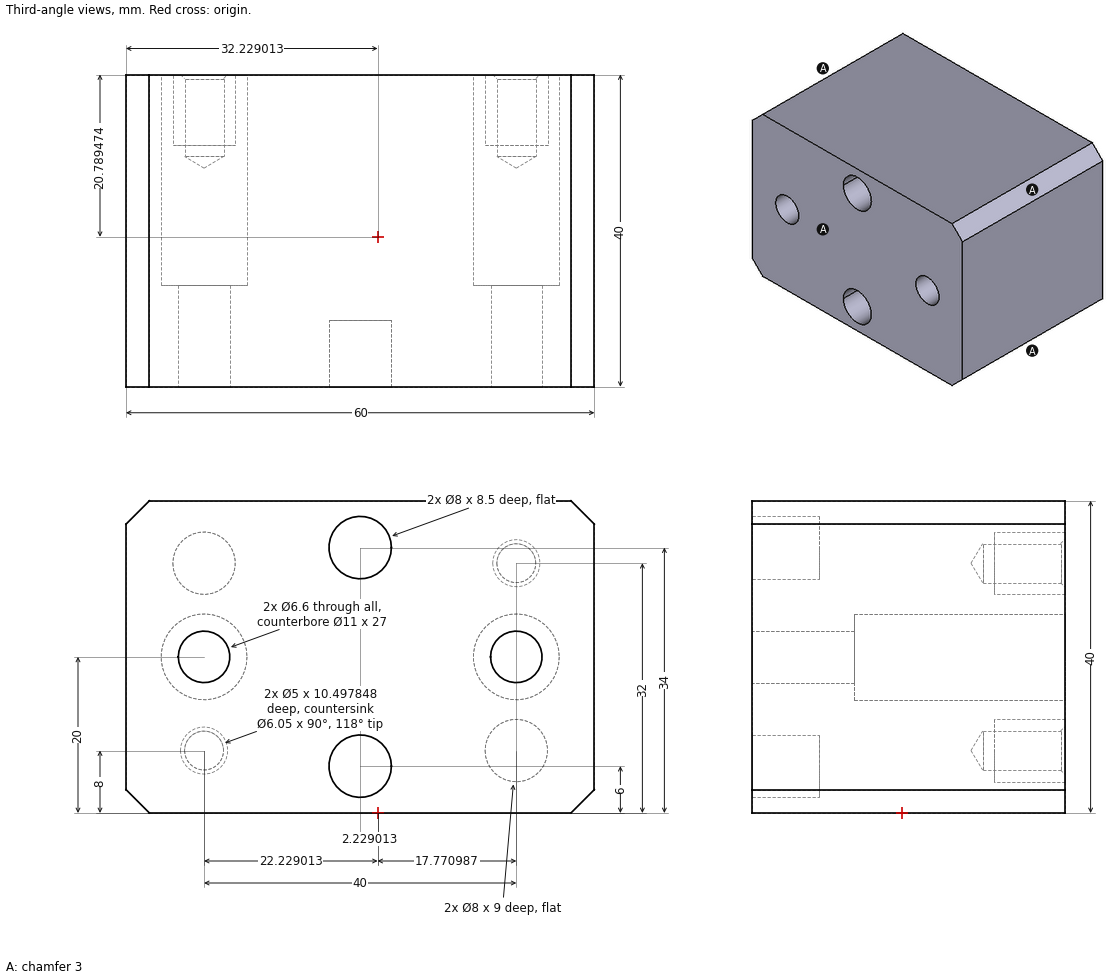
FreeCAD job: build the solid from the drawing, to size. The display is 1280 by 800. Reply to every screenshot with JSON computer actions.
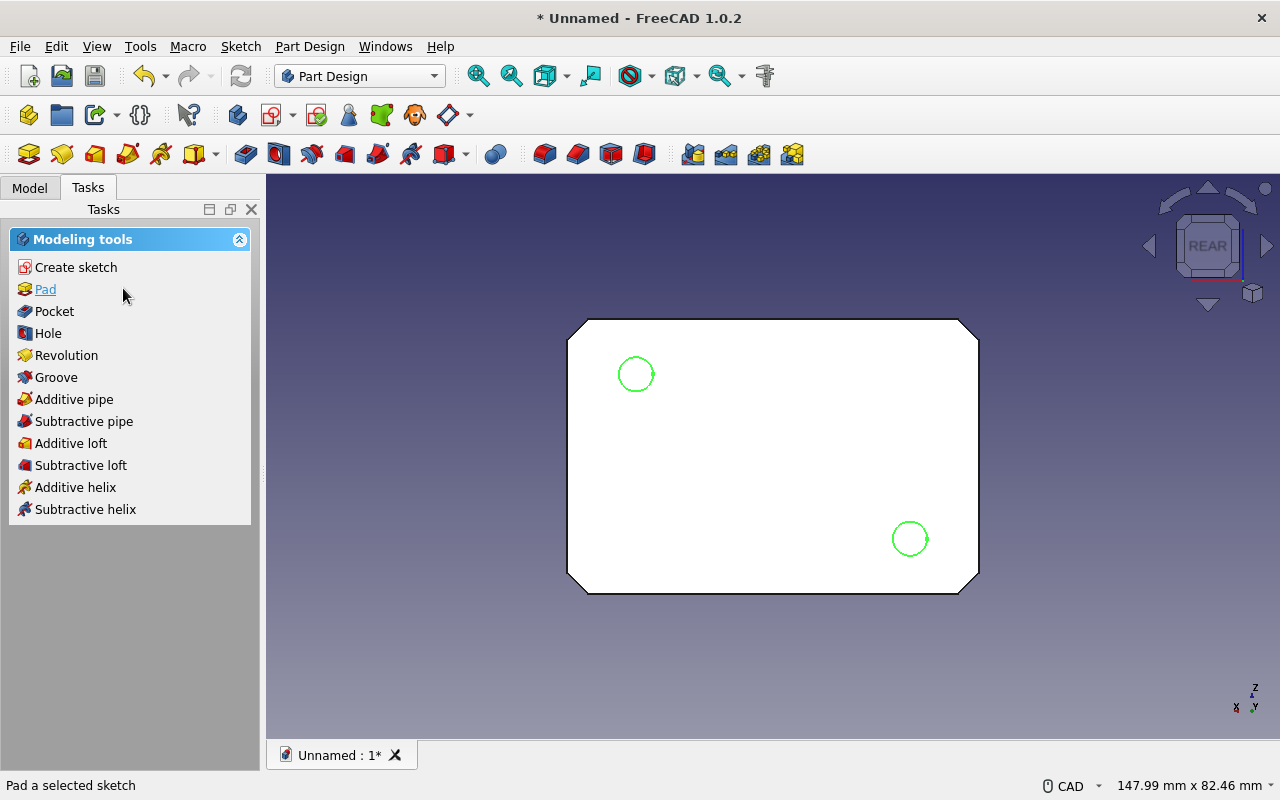
{"action": "left_click", "coordinate": [279, 154]}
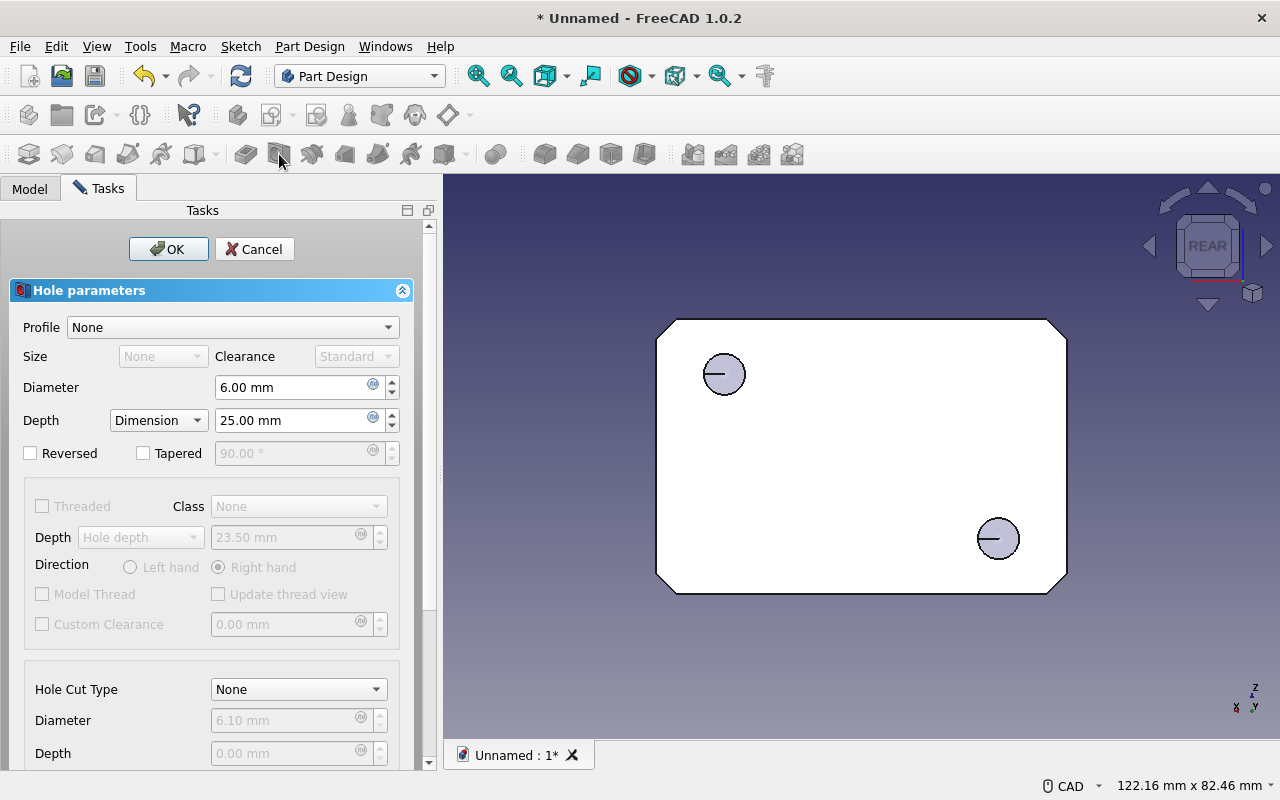
{"action": "triple_click", "coordinate": [300, 388]}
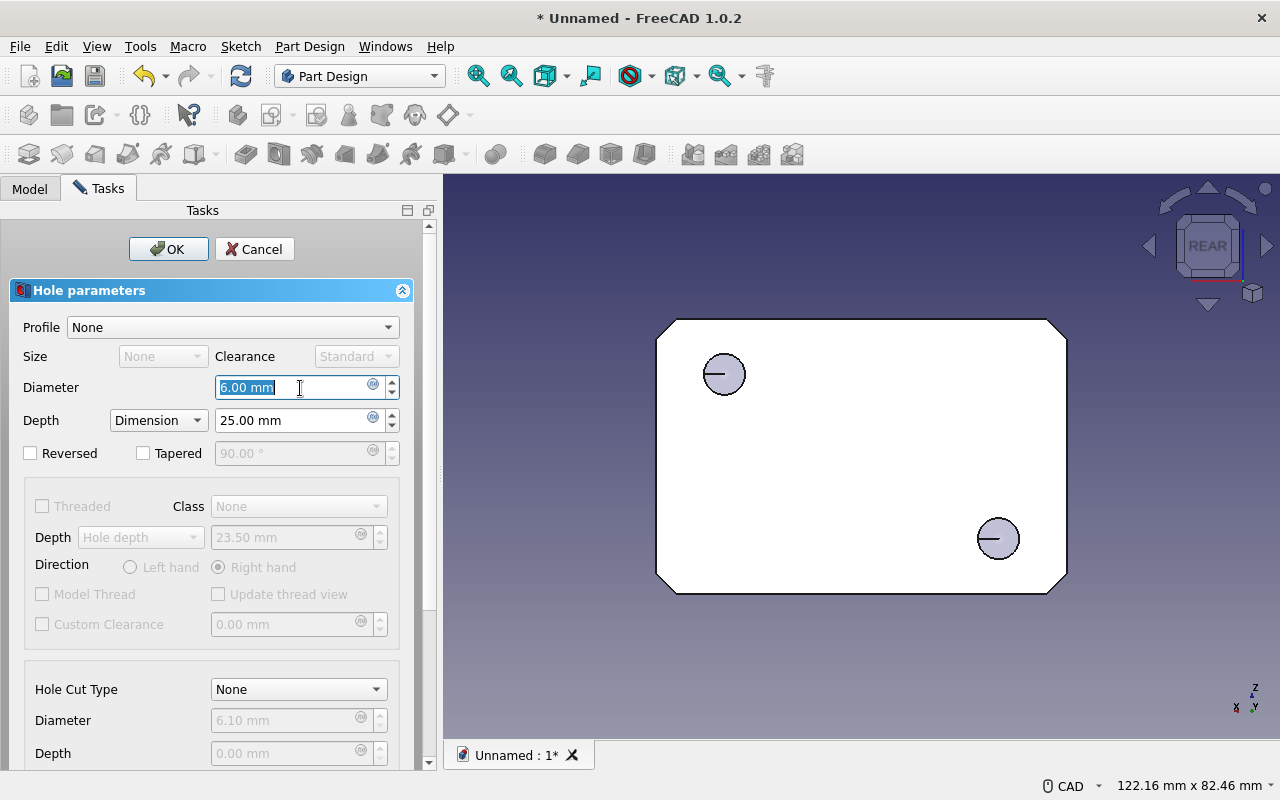
{"action": "type", "text": "5"}
{"action": "key", "text": "Tab"}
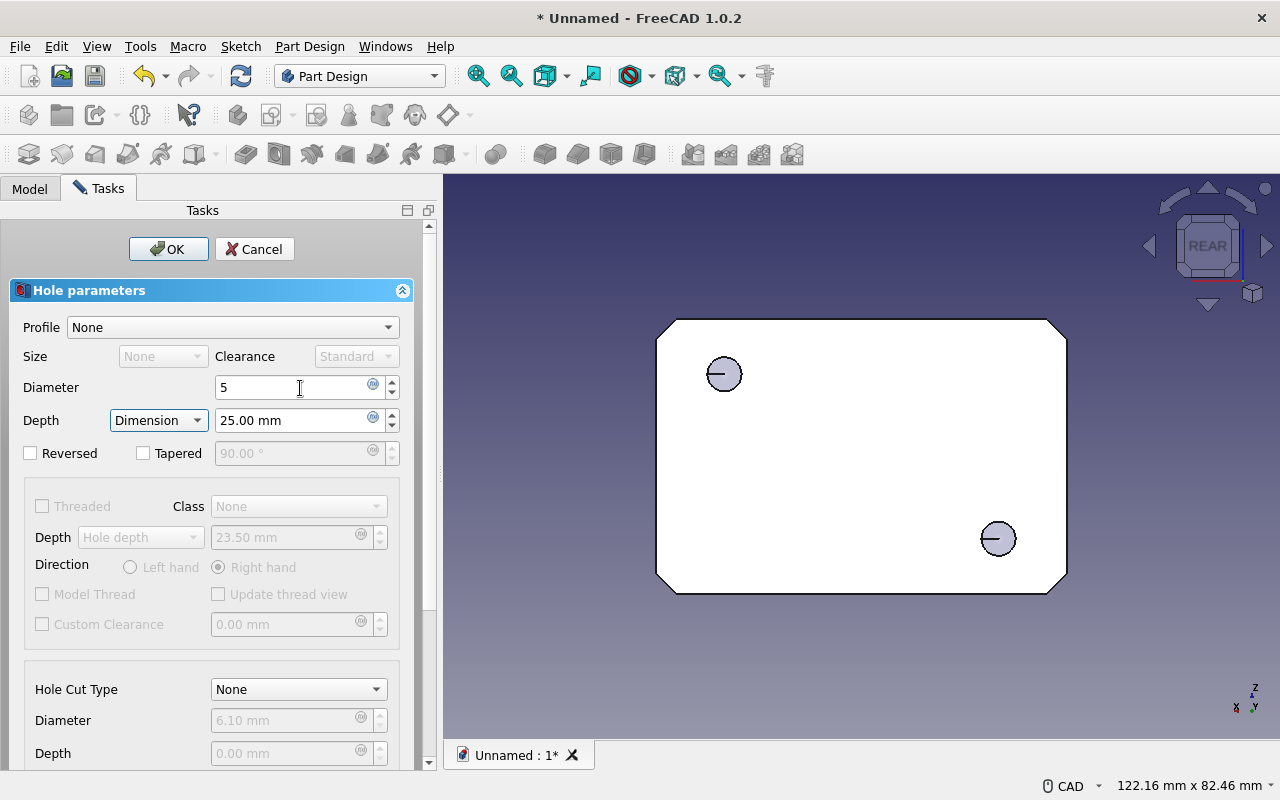
{"action": "triple_click", "coordinate": [300, 420]}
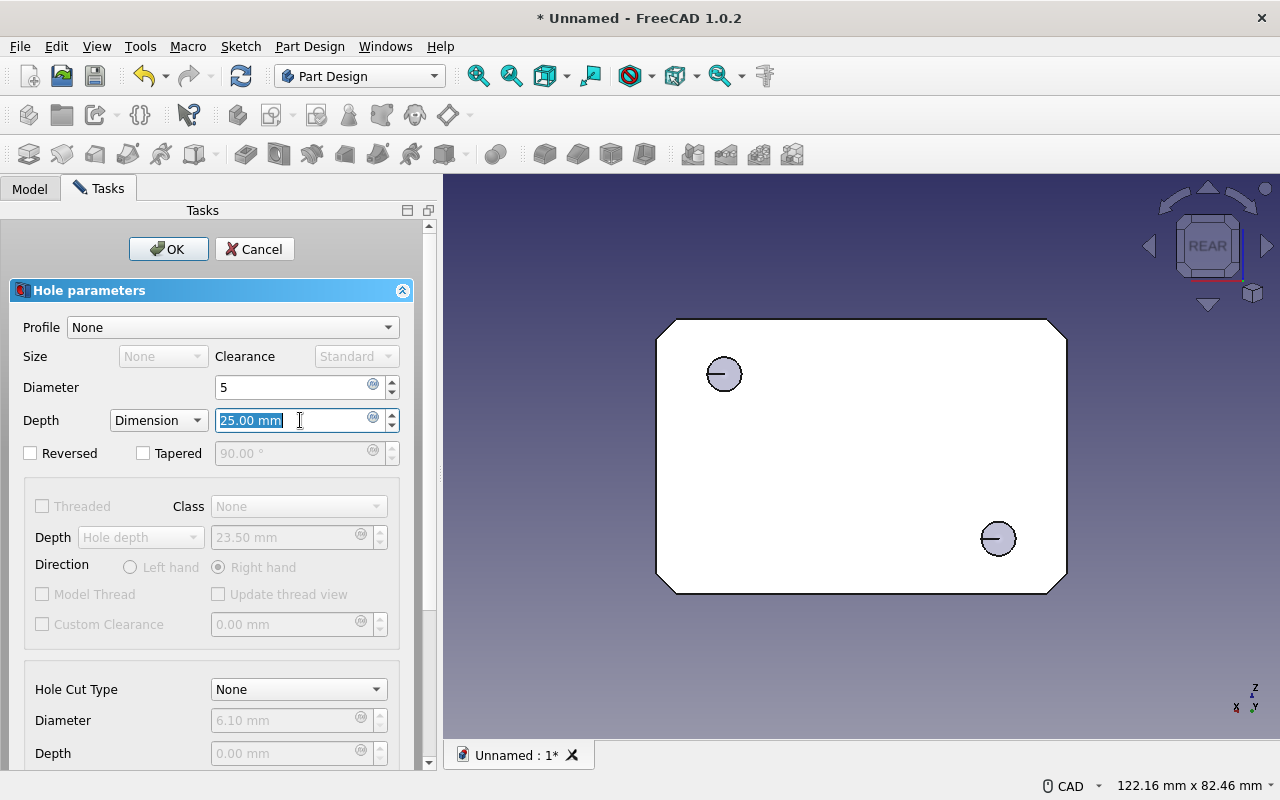
{"action": "type", "text": "10.497848"}
{"action": "key", "text": "Tab"}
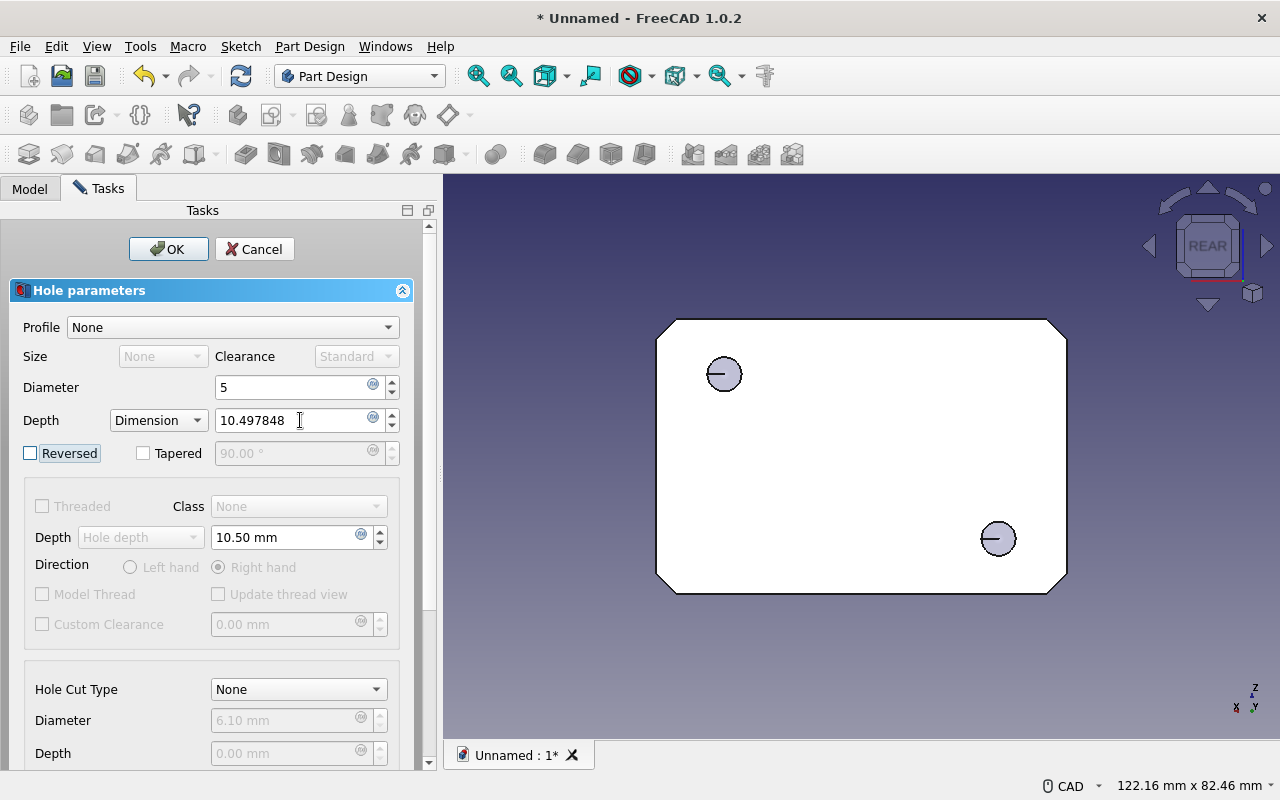
{"action": "left_click", "coordinate": [300, 690]}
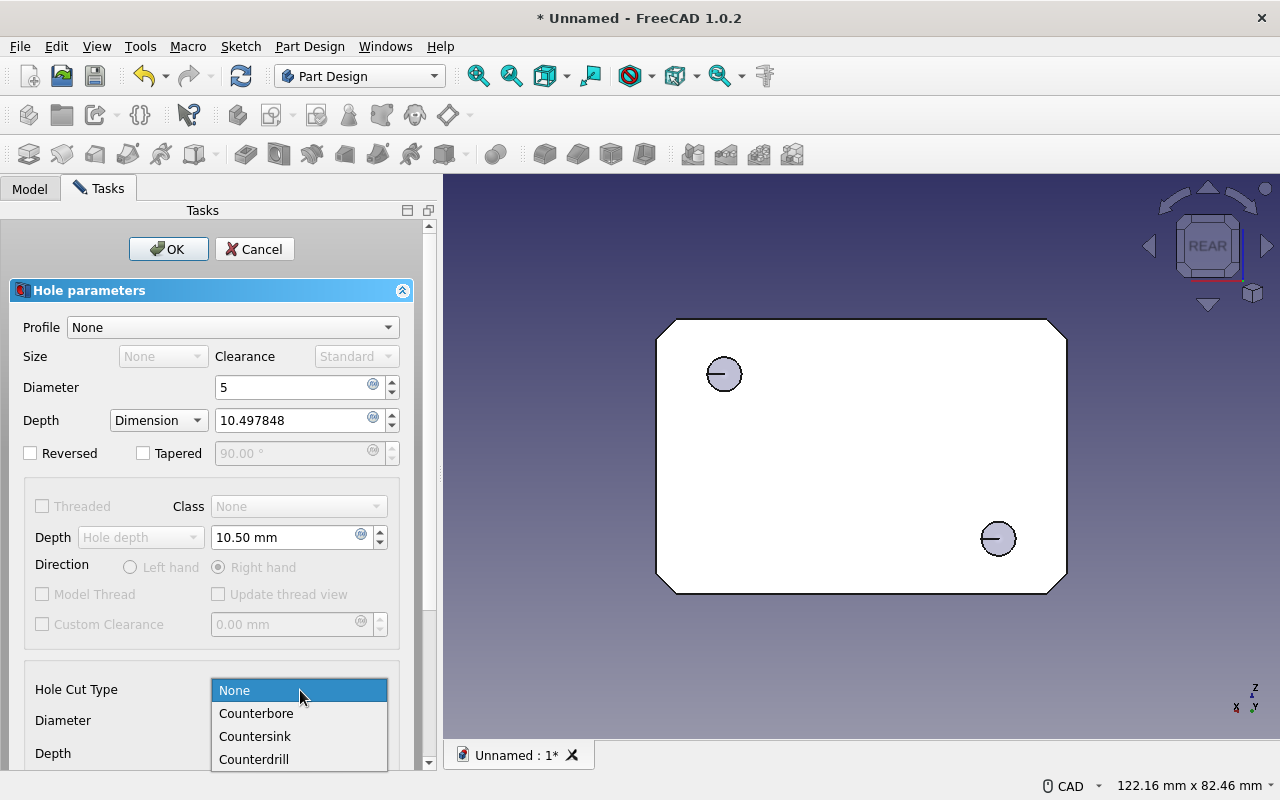
{"action": "left_click", "coordinate": [298, 736]}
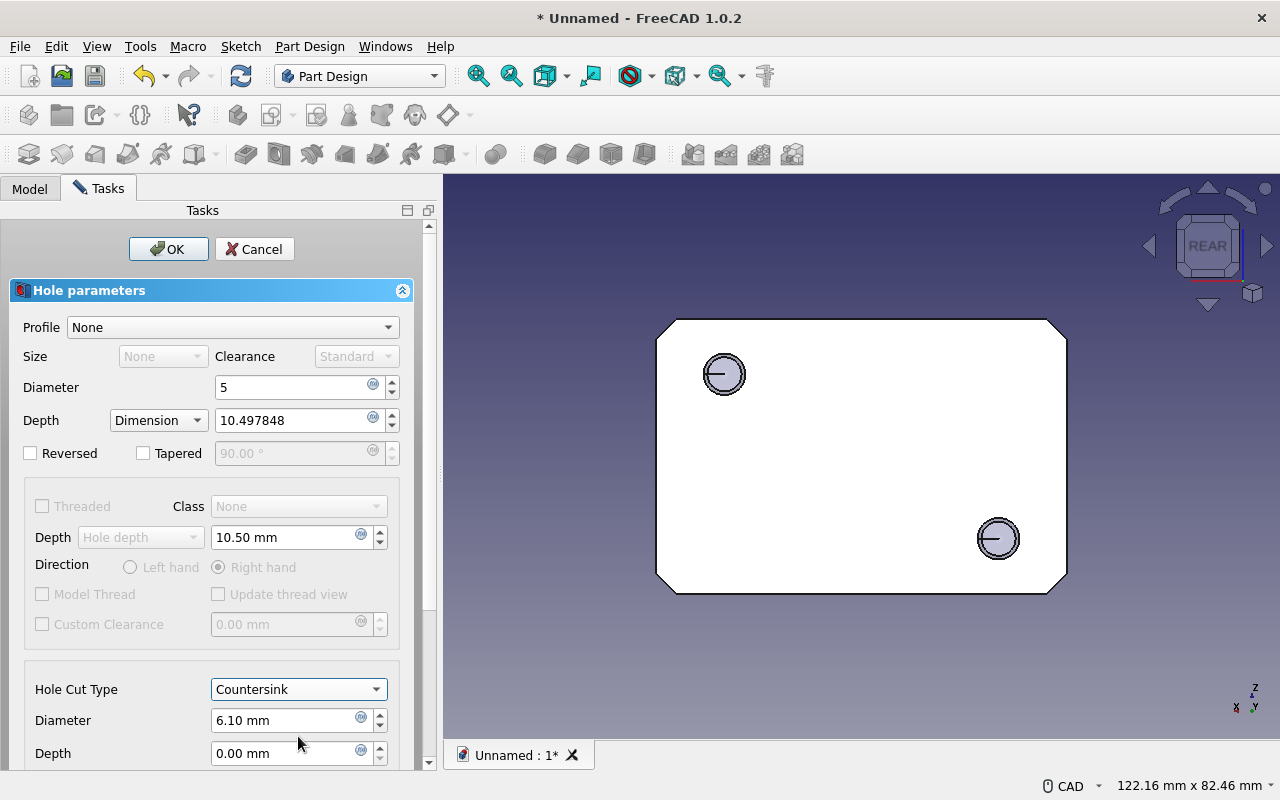
{"action": "triple_click", "coordinate": [292, 720]}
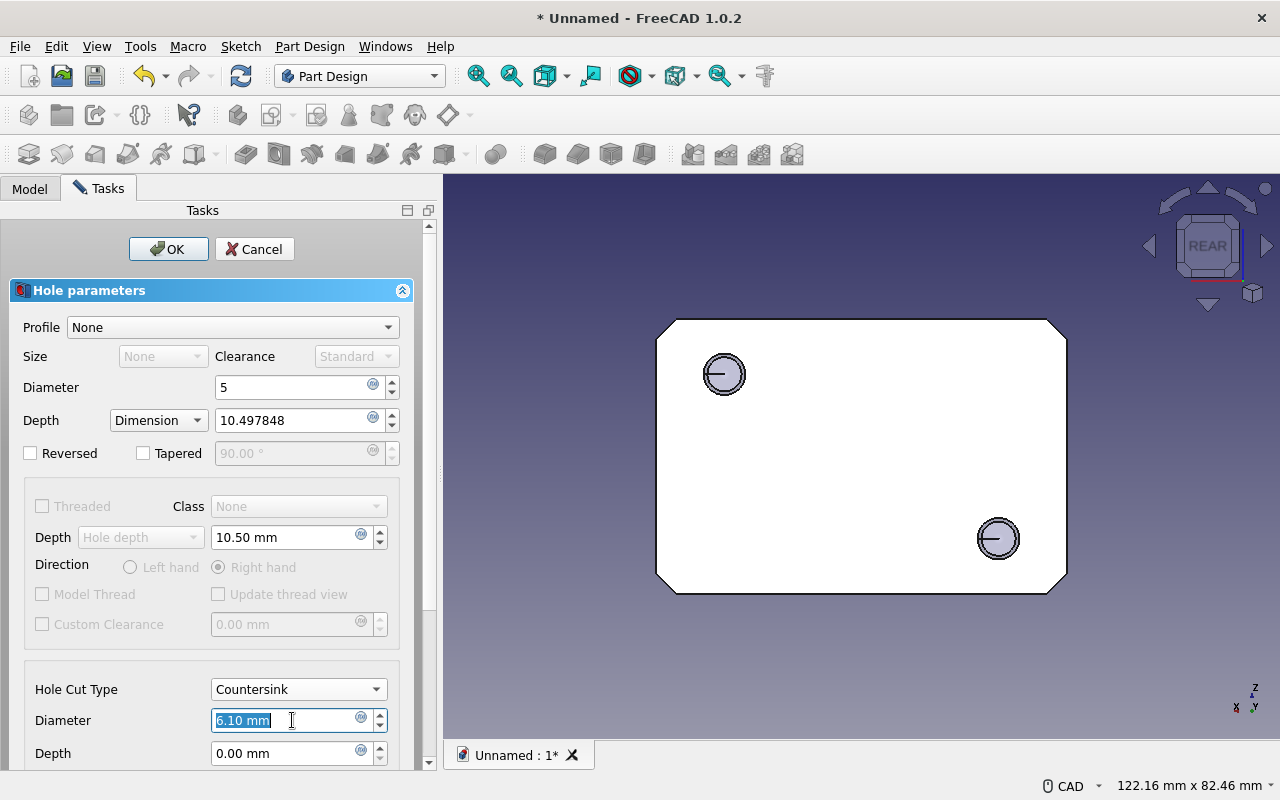
{"action": "type", "text": "6.05"}
{"action": "key", "text": "Tab"}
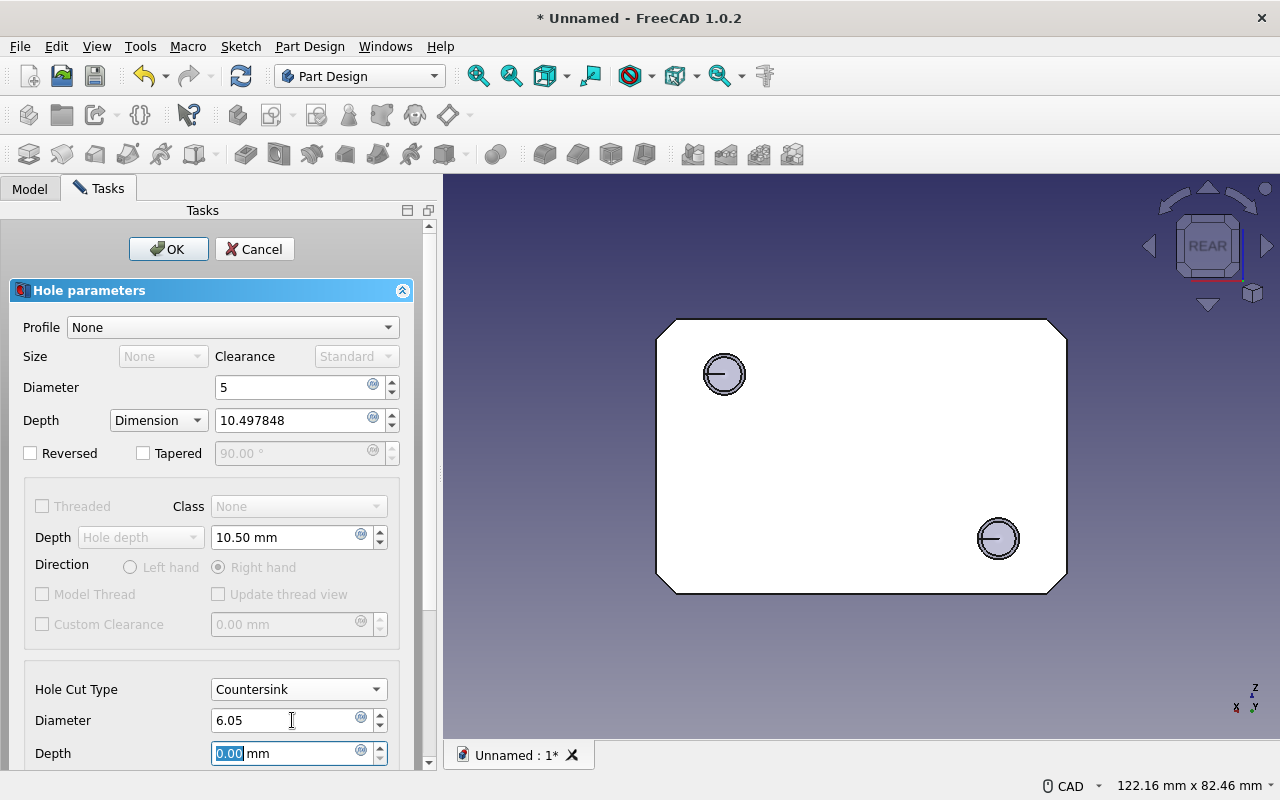
{"action": "left_click", "coordinate": [169, 249]}